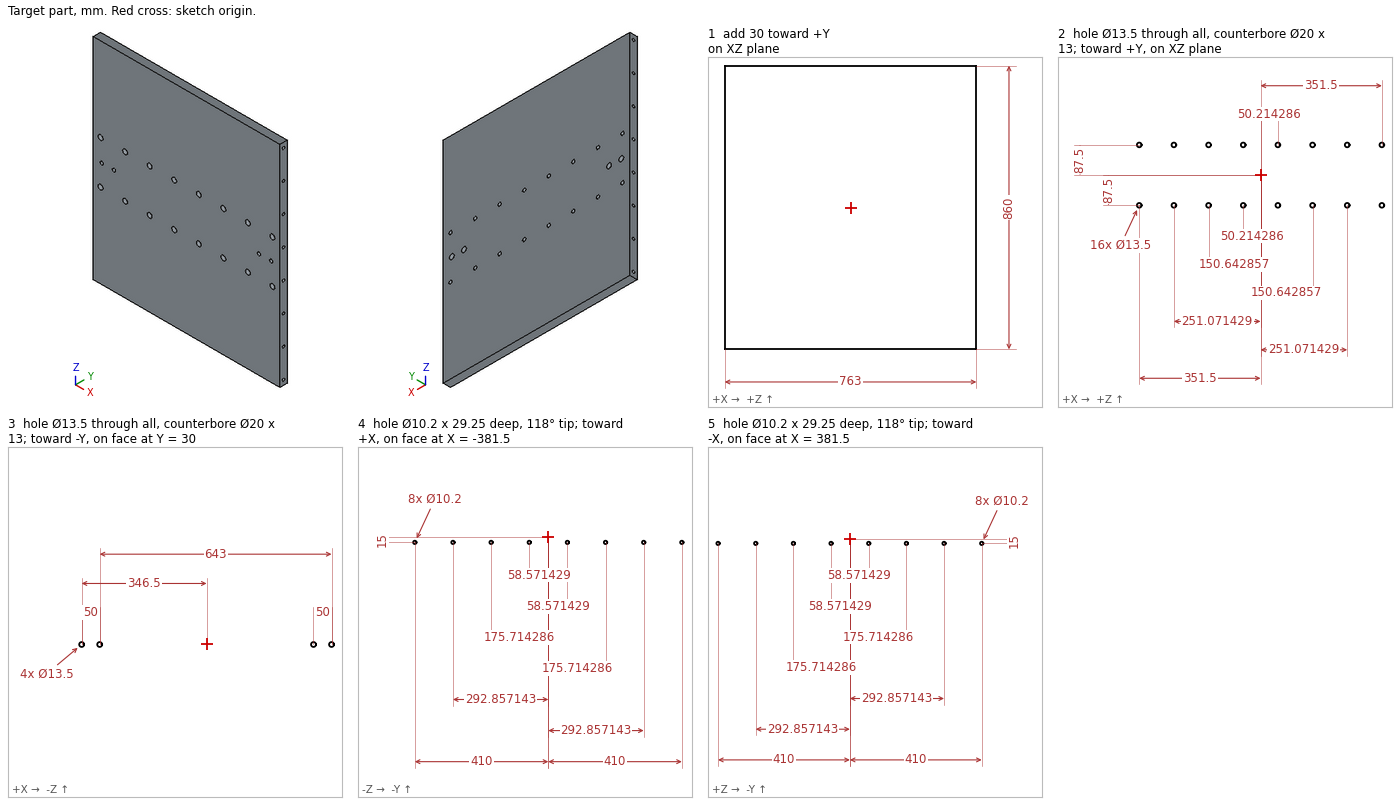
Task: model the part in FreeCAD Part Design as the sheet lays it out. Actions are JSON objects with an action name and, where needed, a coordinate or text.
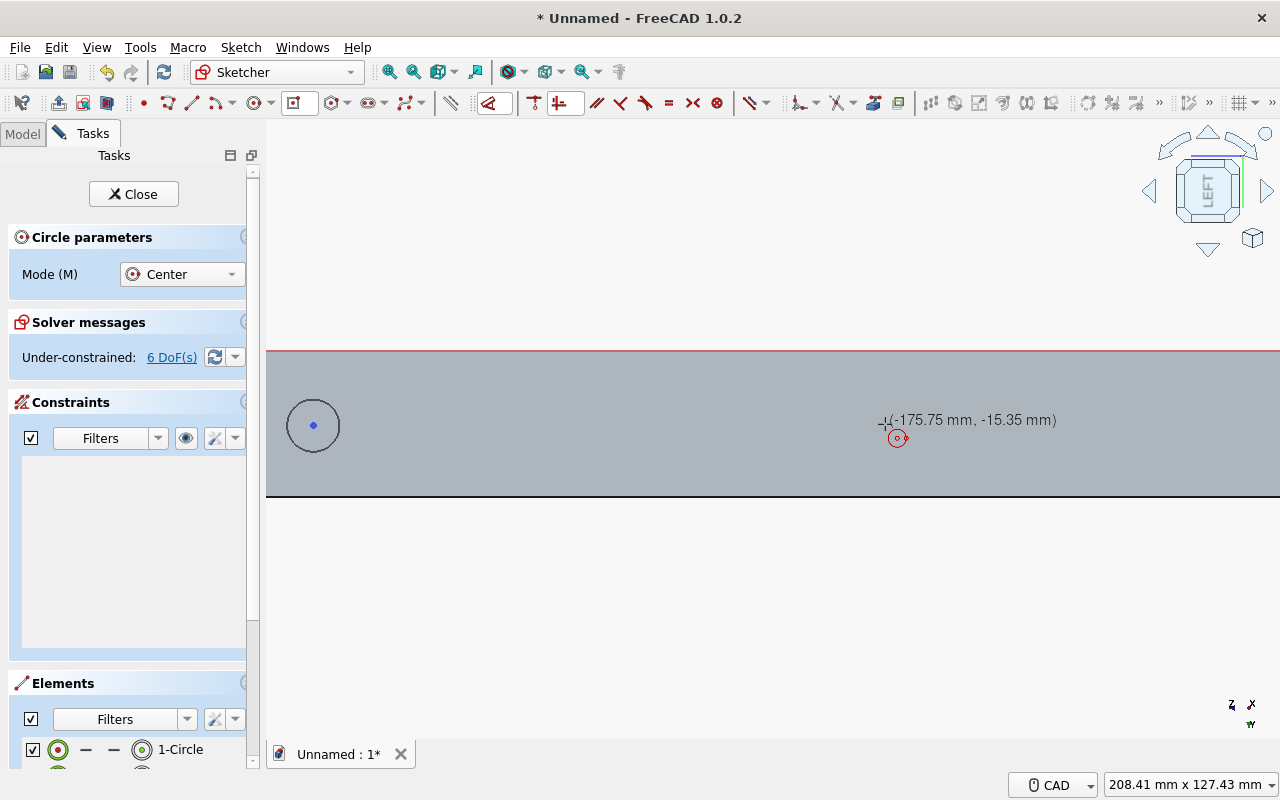
{"action": "scroll", "coordinate": [542, 434], "scroll_direction": "down", "scroll_amount": 10}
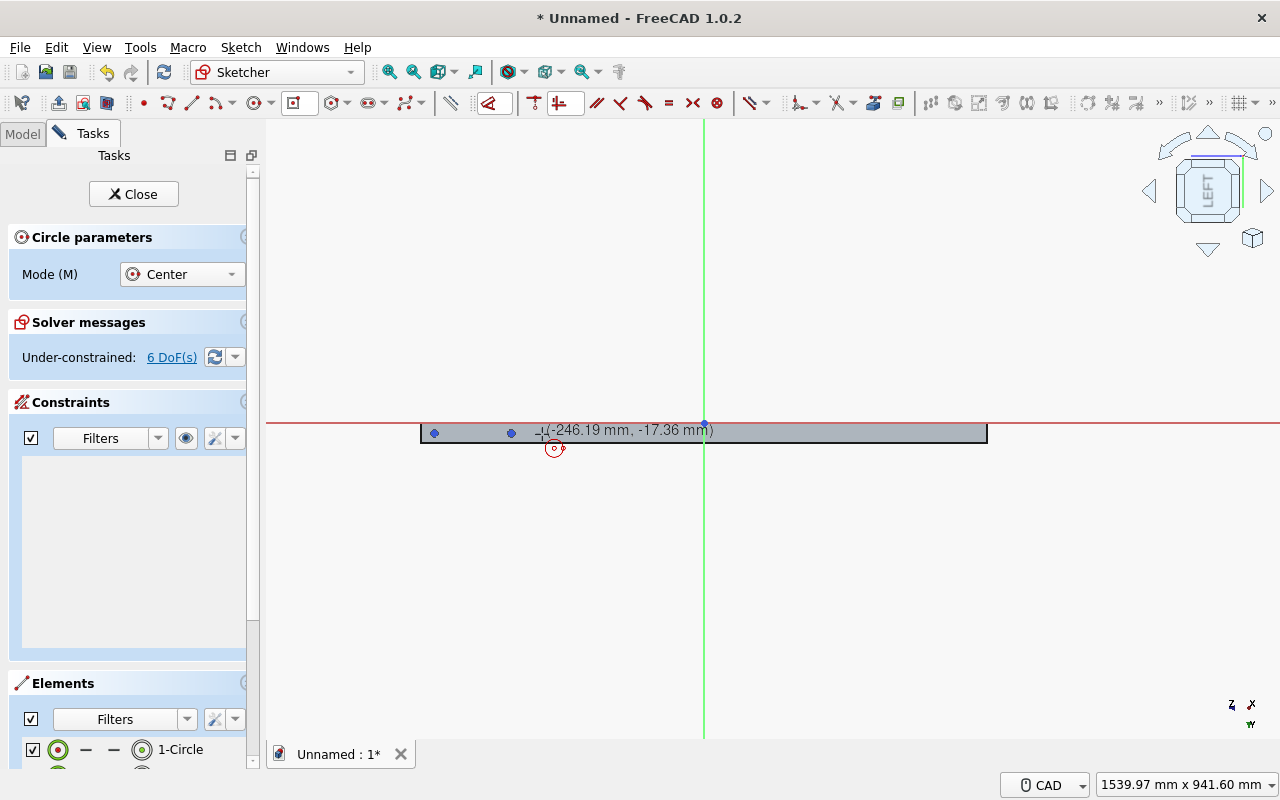
{"action": "scroll", "coordinate": [589, 433], "scroll_direction": "up", "scroll_amount": 3}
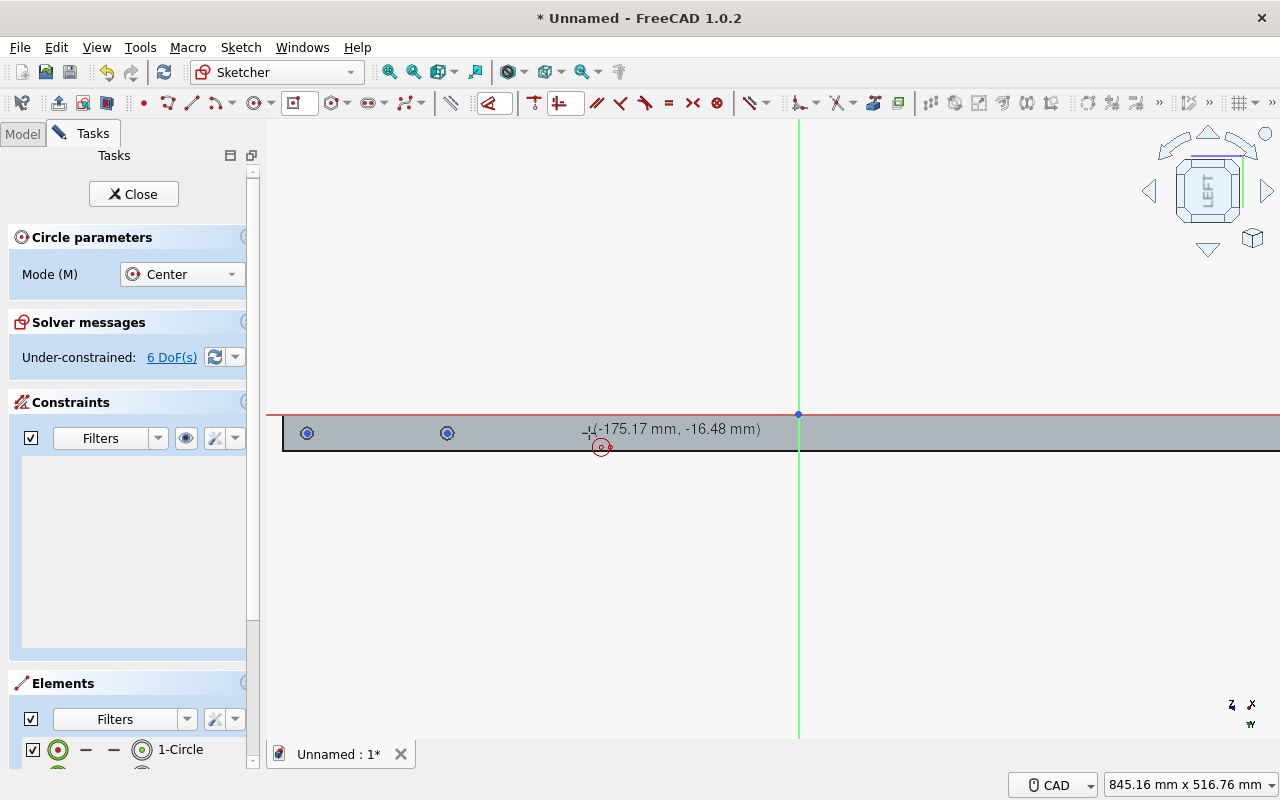
{"action": "left_click", "coordinate": [588, 433]}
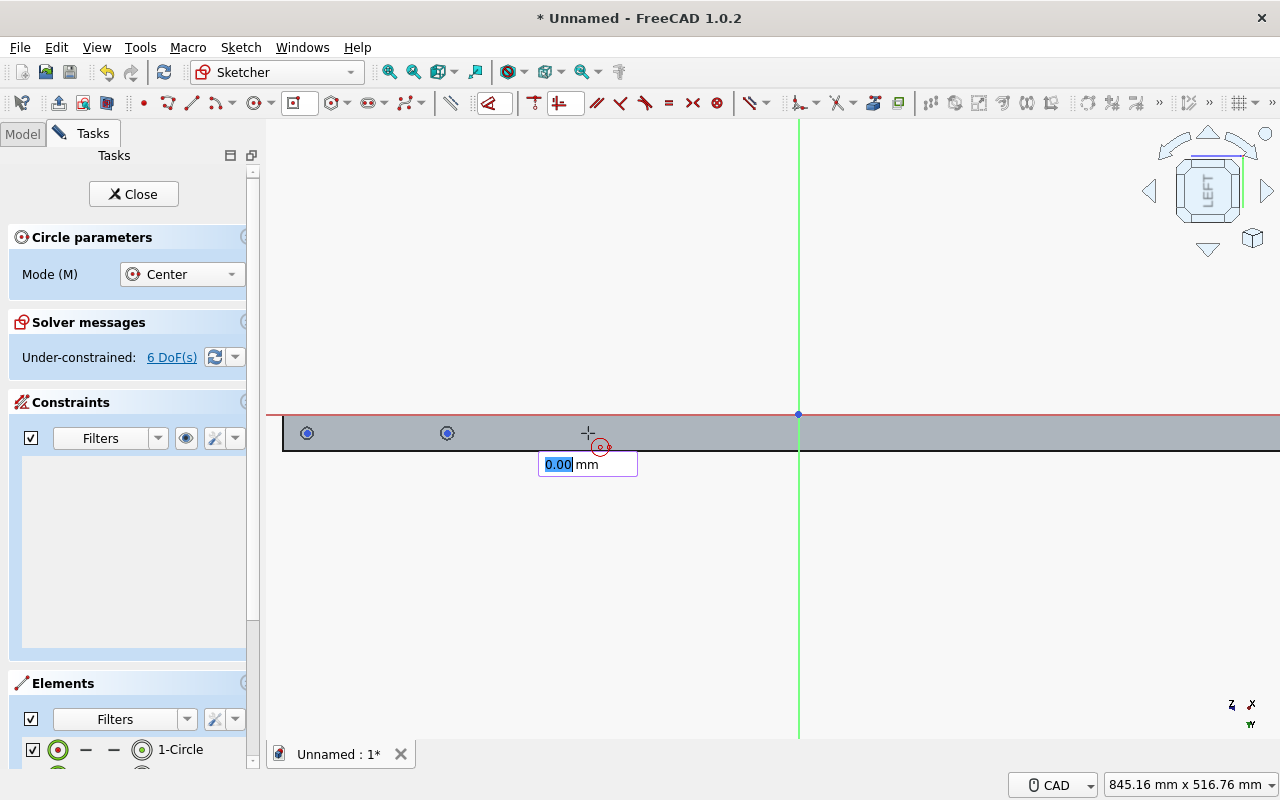
{"action": "scroll", "coordinate": [592, 437], "scroll_direction": "up", "scroll_amount": 5}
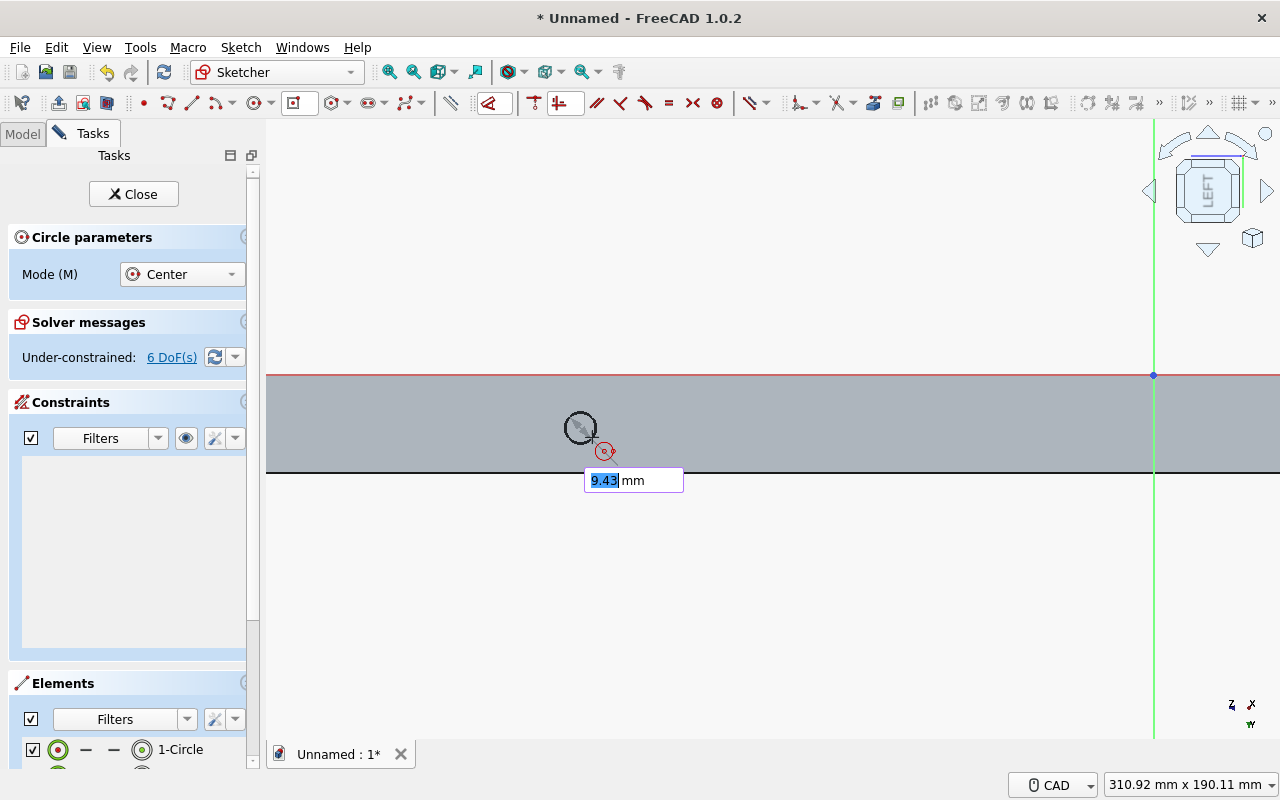
{"action": "left_click", "coordinate": [593, 436]}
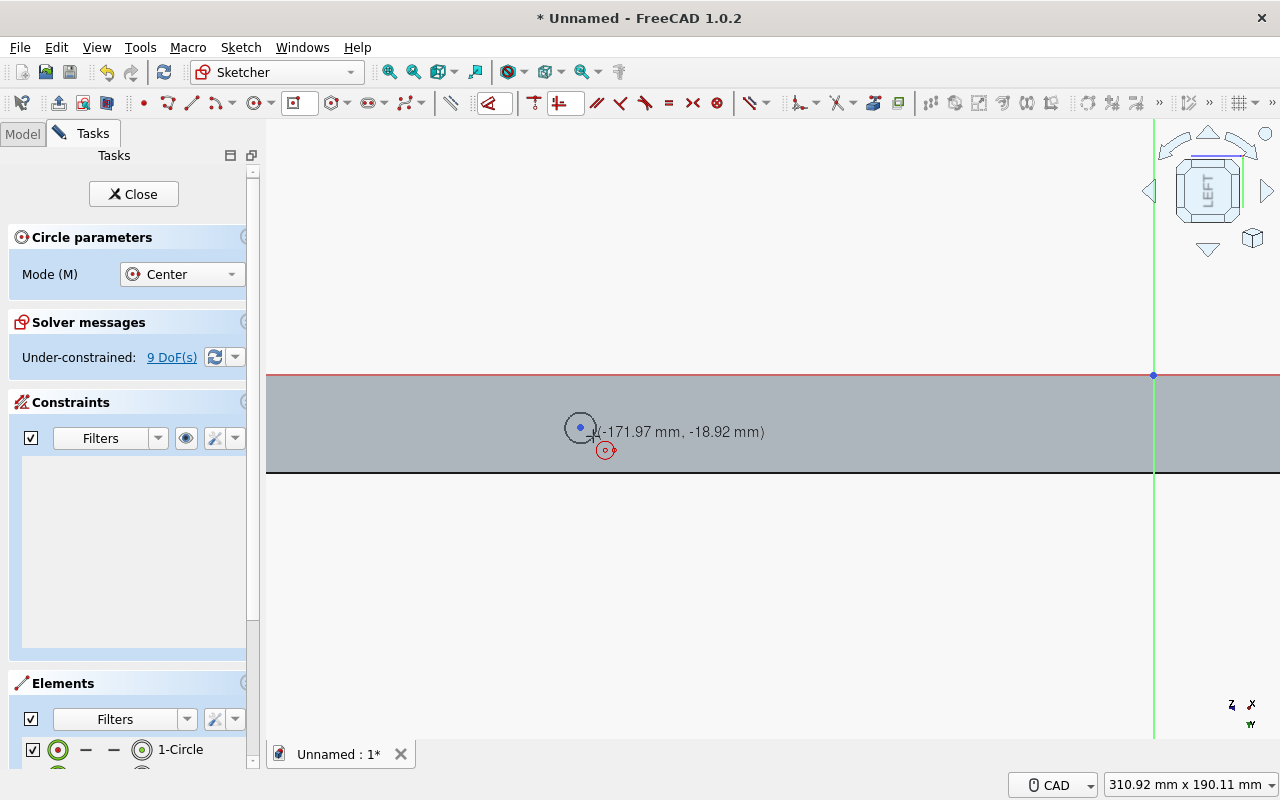
{"action": "scroll", "coordinate": [963, 424], "scroll_direction": "up", "scroll_amount": 2}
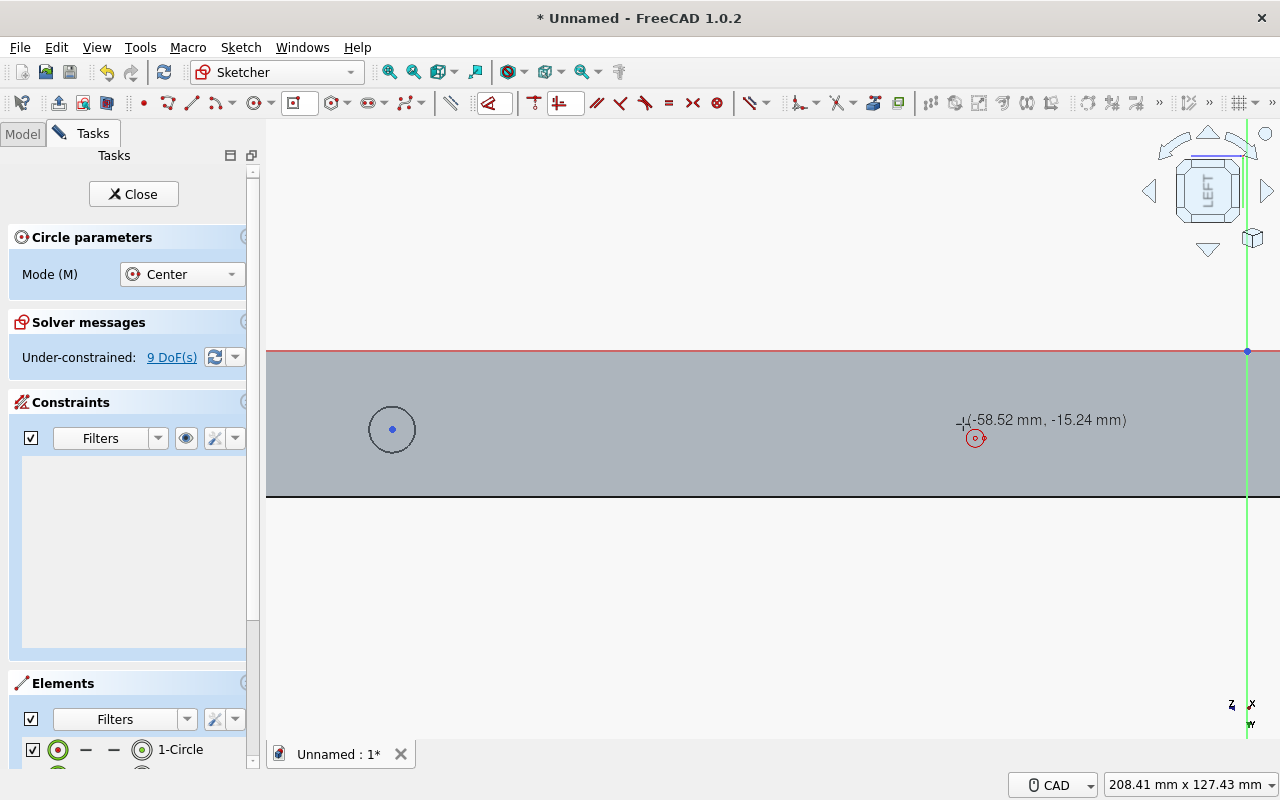
{"action": "scroll", "coordinate": [620, 434], "scroll_direction": "down", "scroll_amount": 10}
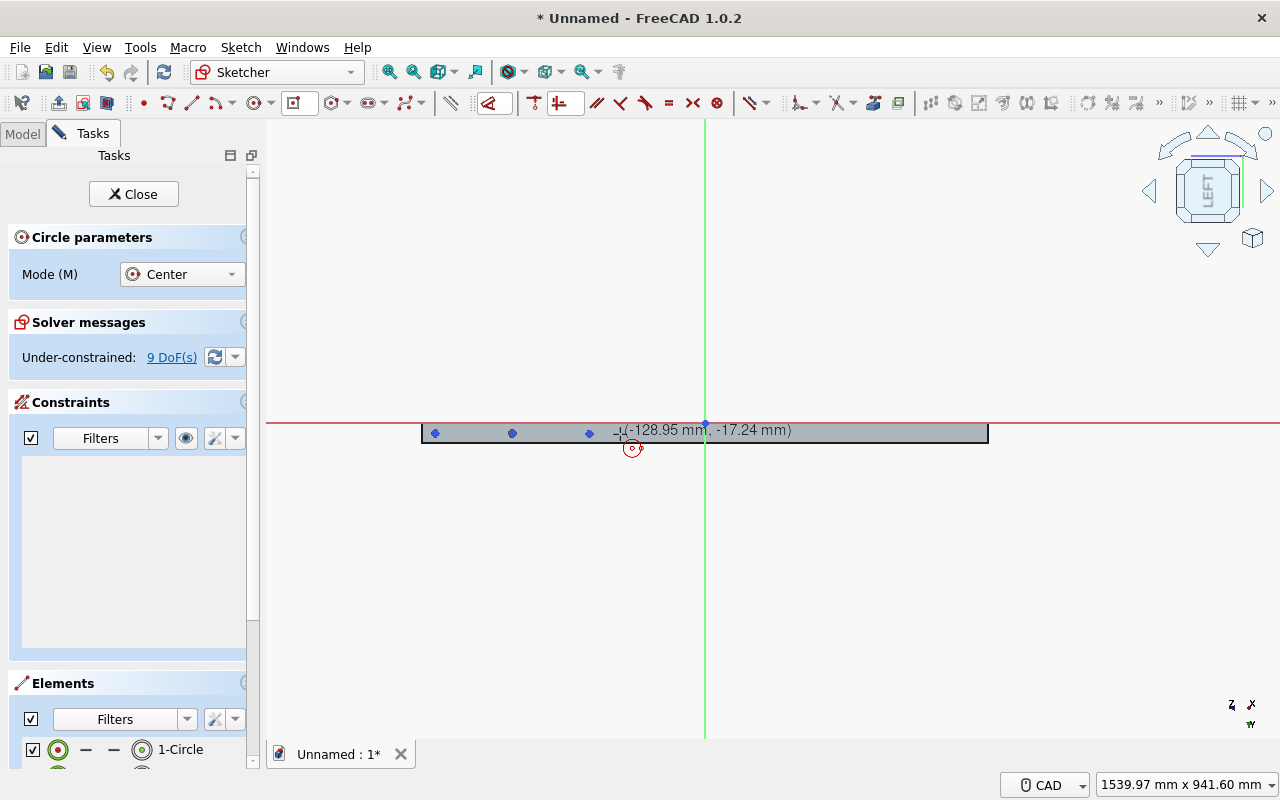
{"action": "scroll", "coordinate": [667, 433], "scroll_direction": "up", "scroll_amount": 3}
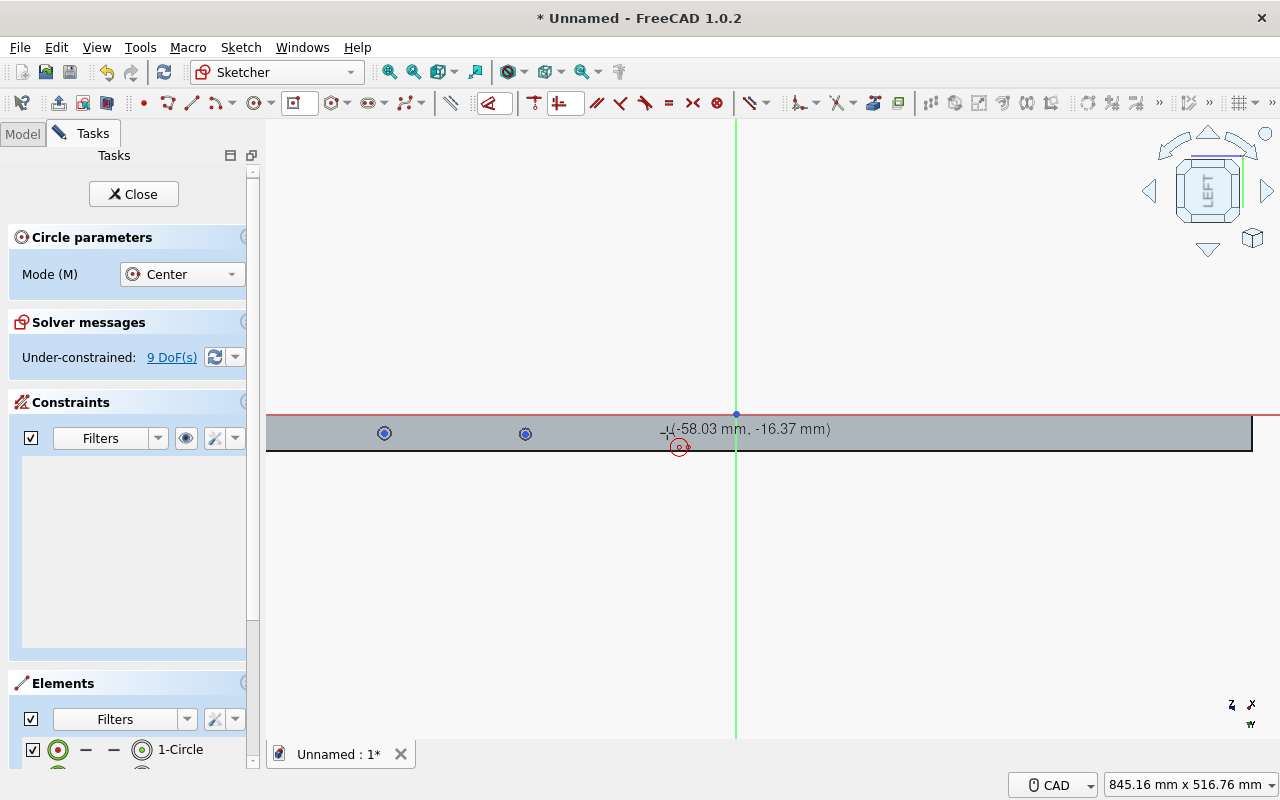
{"action": "left_click", "coordinate": [666, 433]}